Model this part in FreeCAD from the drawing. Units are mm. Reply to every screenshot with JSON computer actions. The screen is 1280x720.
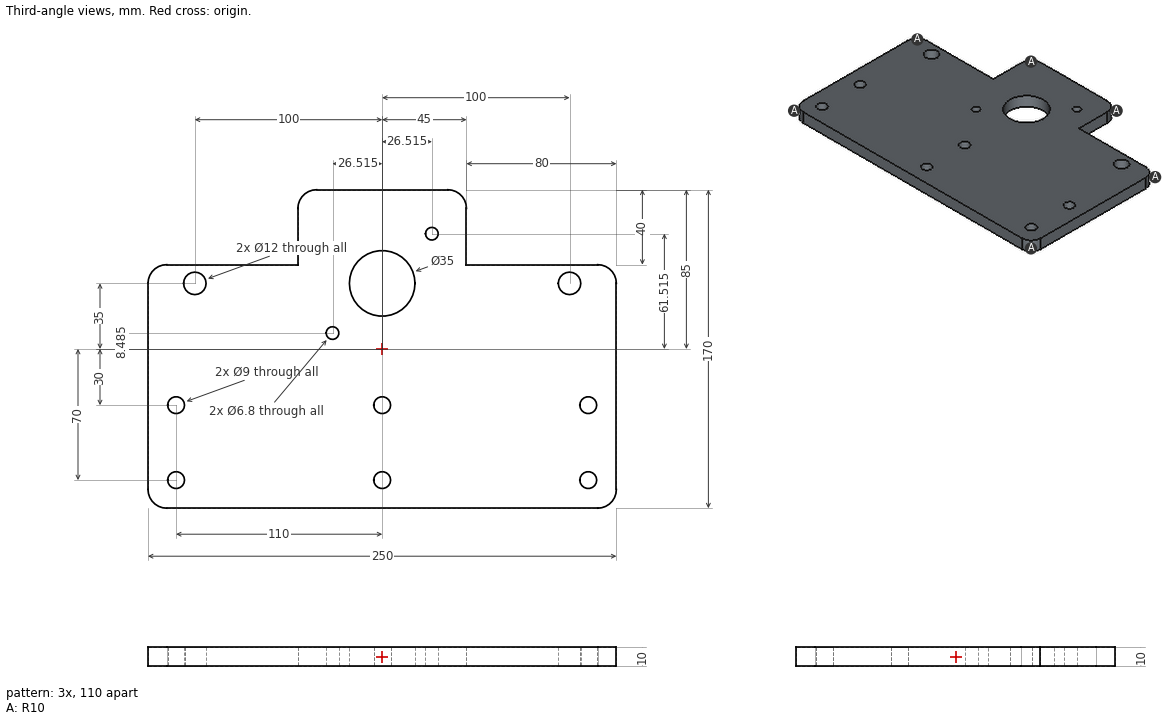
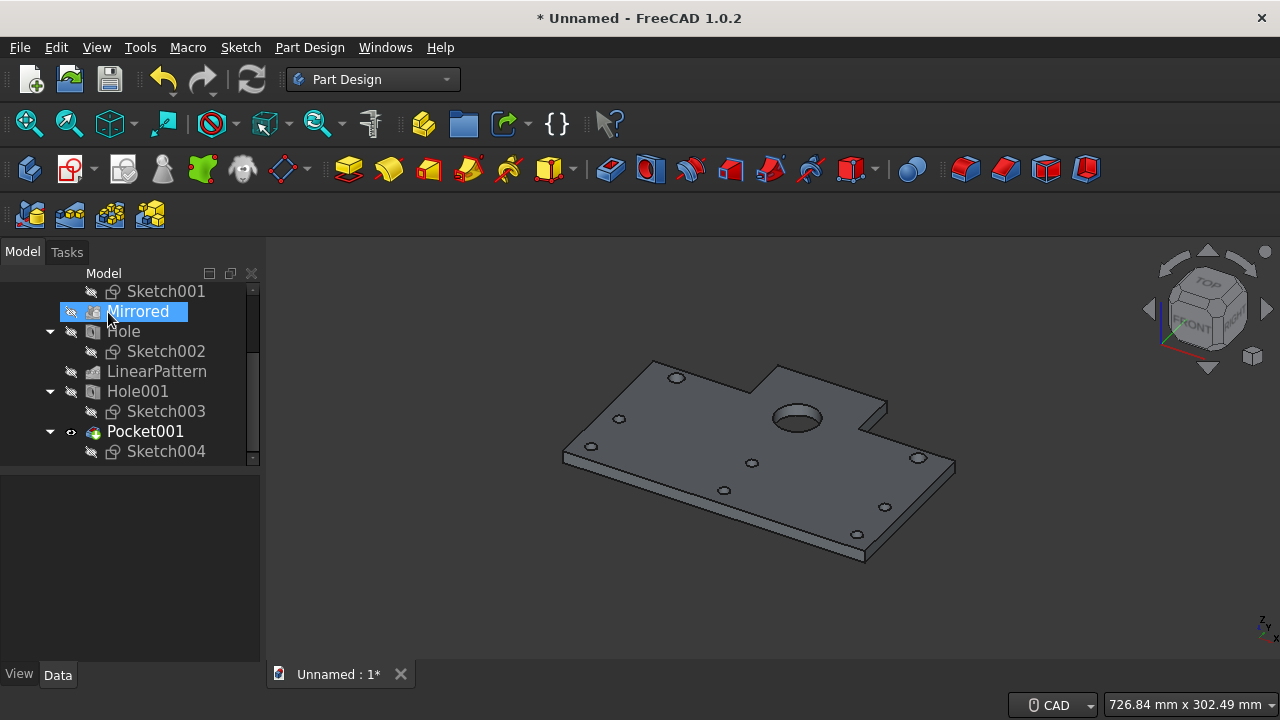
{"action": "left_click", "coordinate": [859, 470]}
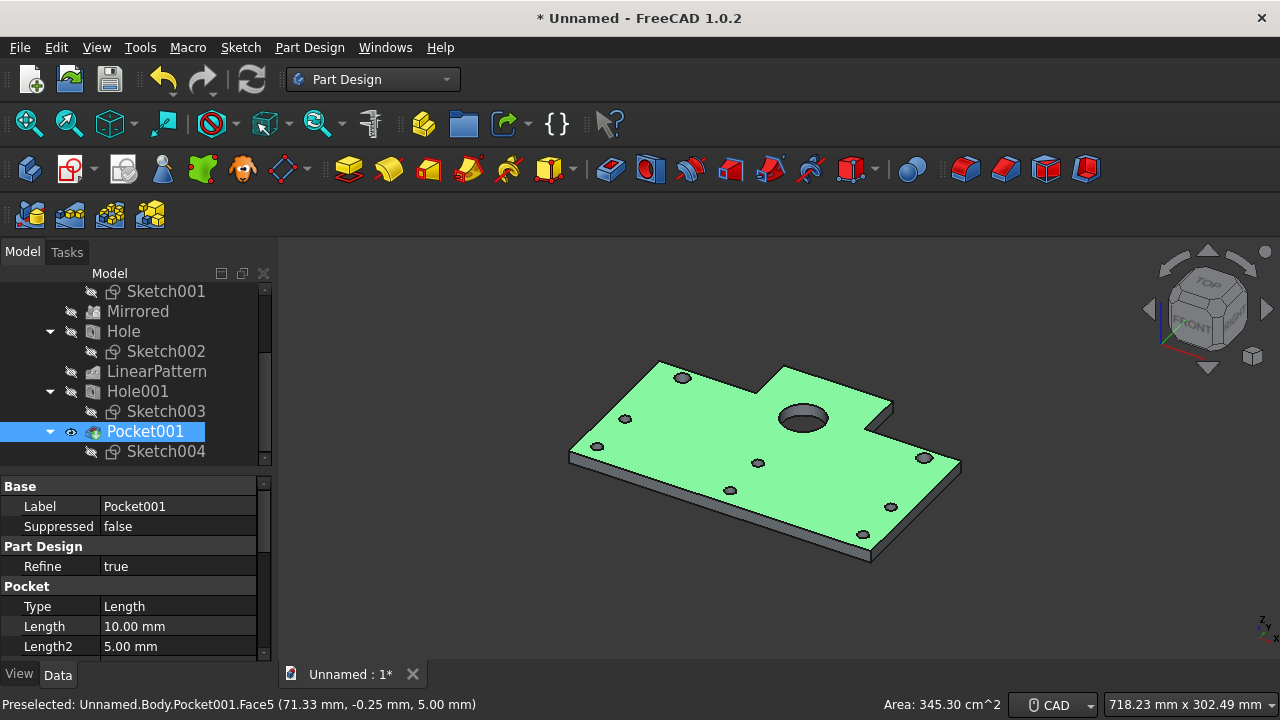
{"action": "left_click", "coordinate": [70, 170]}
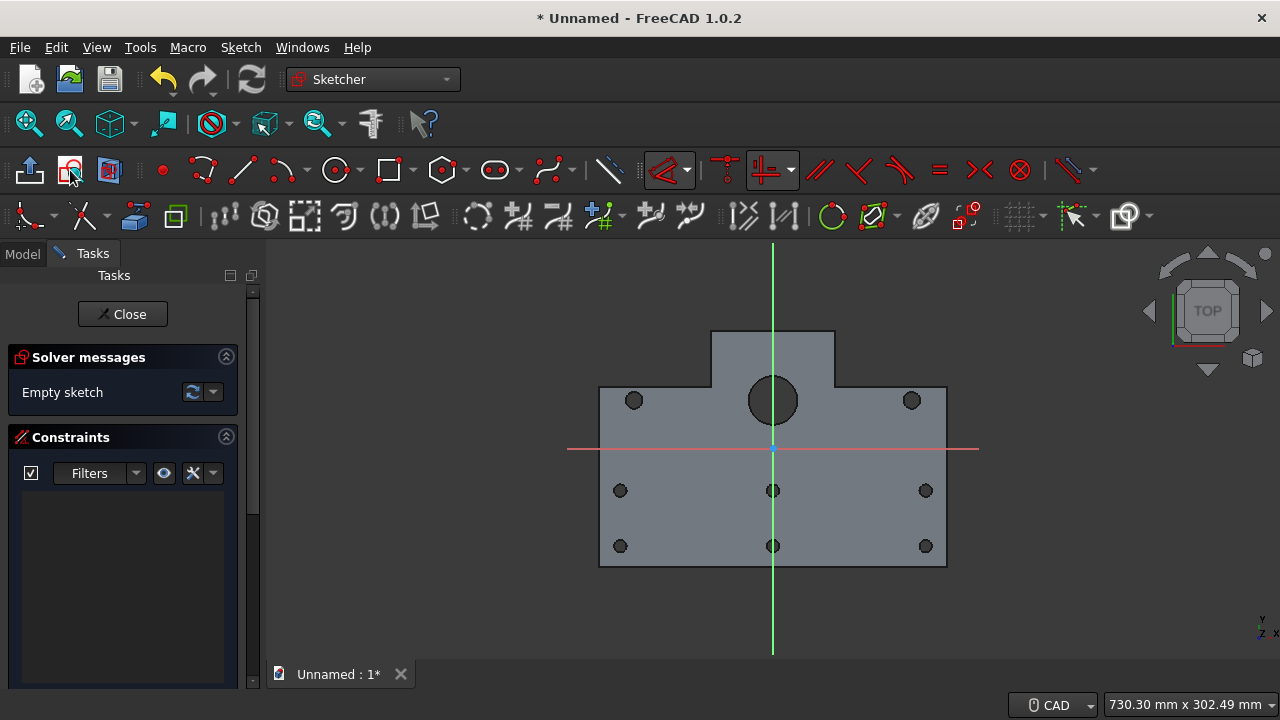
{"action": "scroll", "coordinate": [813, 378], "scroll_direction": "up", "scroll_amount": 5}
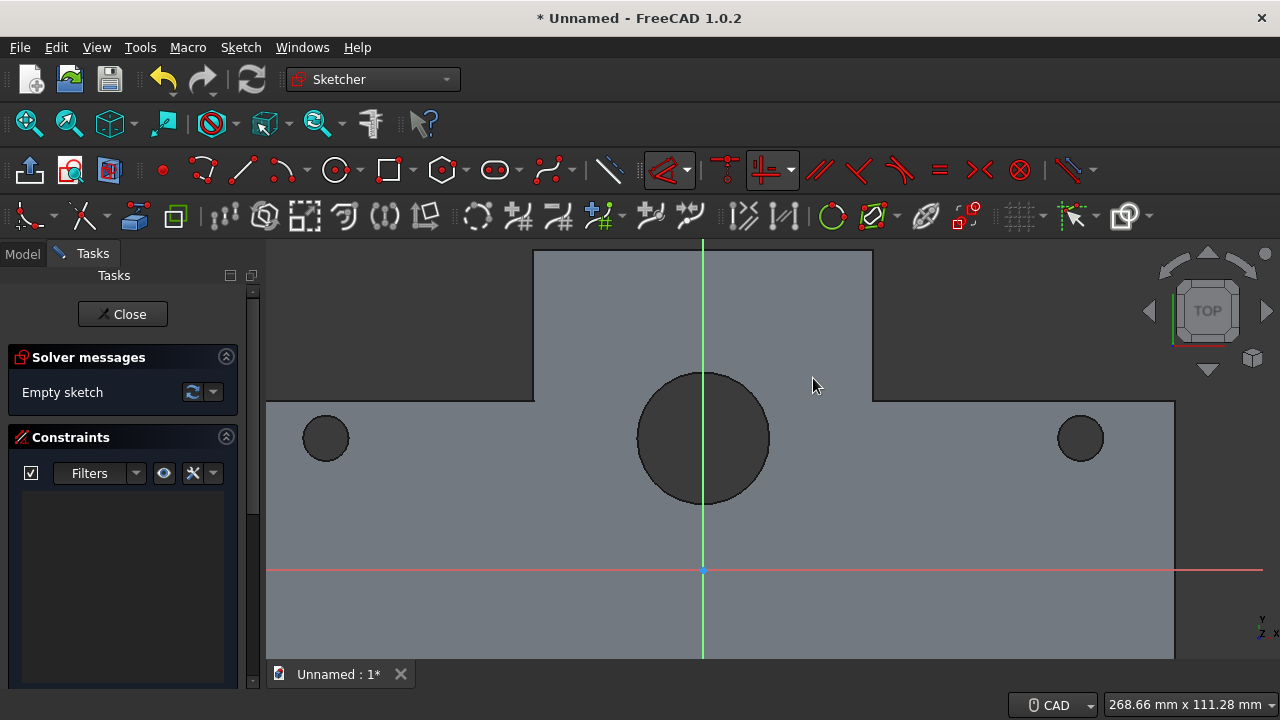
{"action": "left_click", "coordinate": [336, 170]}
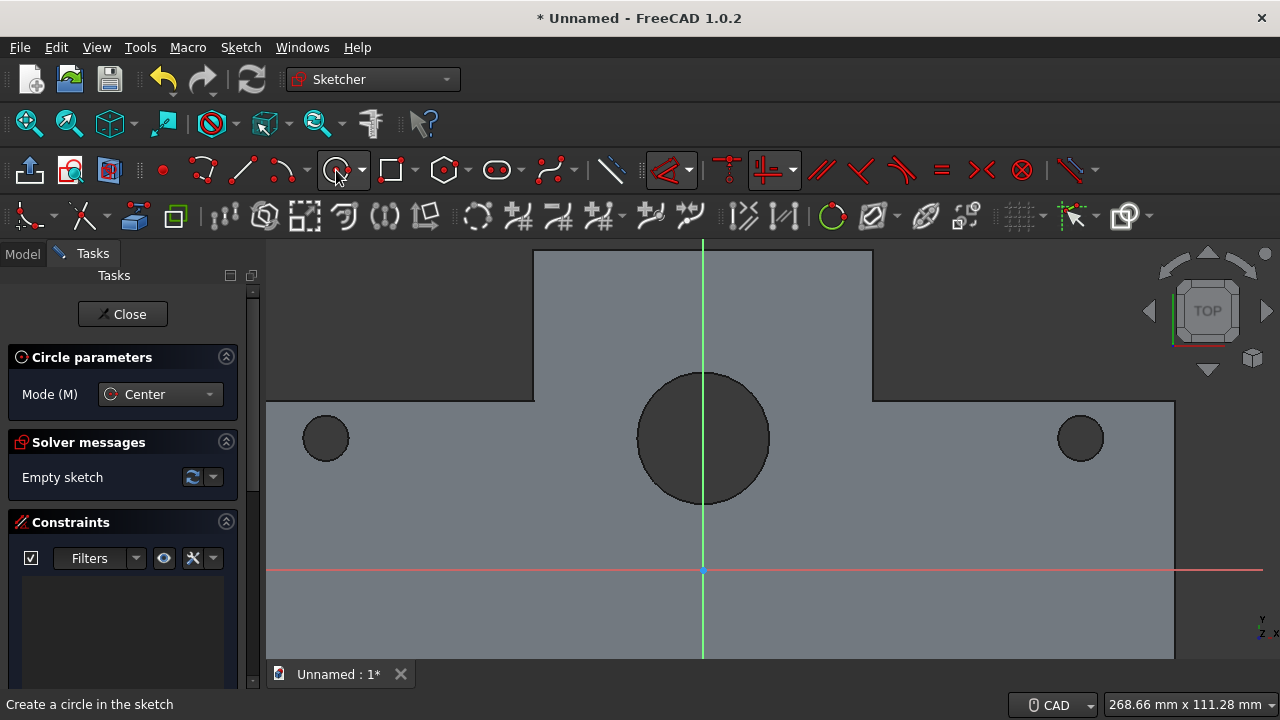
{"action": "scroll", "coordinate": [603, 538], "scroll_direction": "up", "scroll_amount": 3}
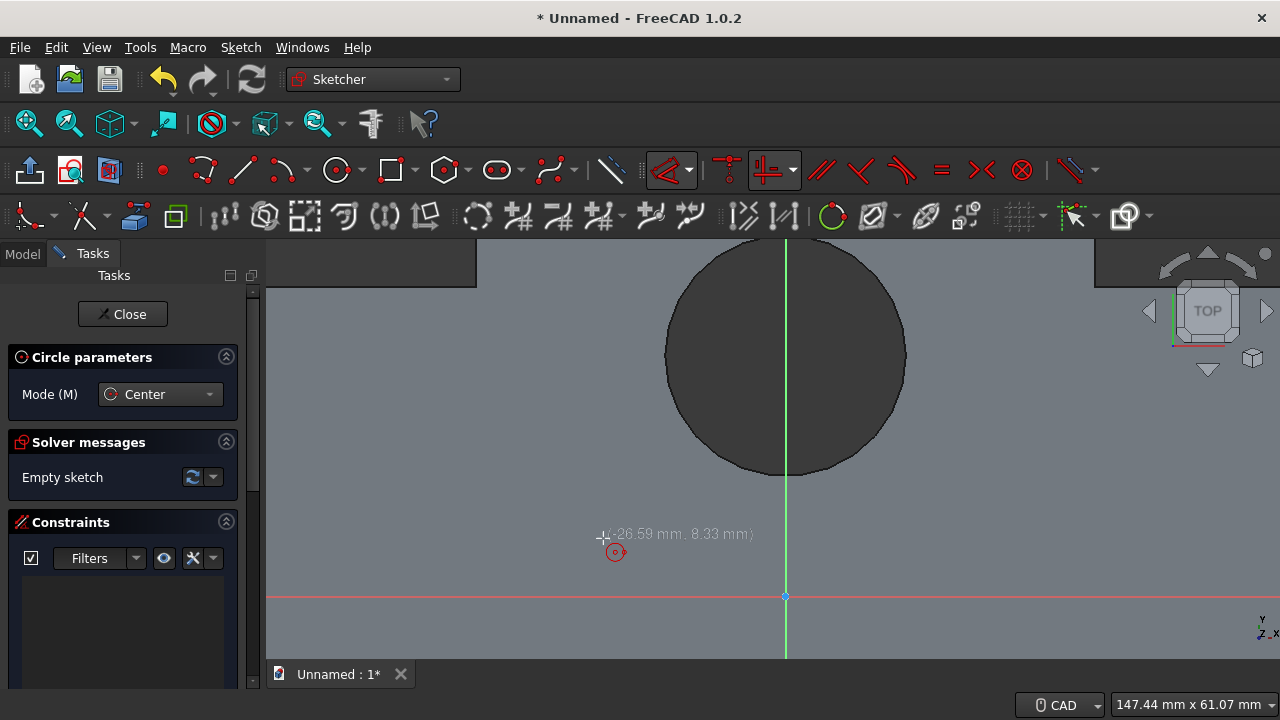
{"action": "left_click", "coordinate": [603, 538]}
{"action": "mouse_move", "coordinate": [620, 522]}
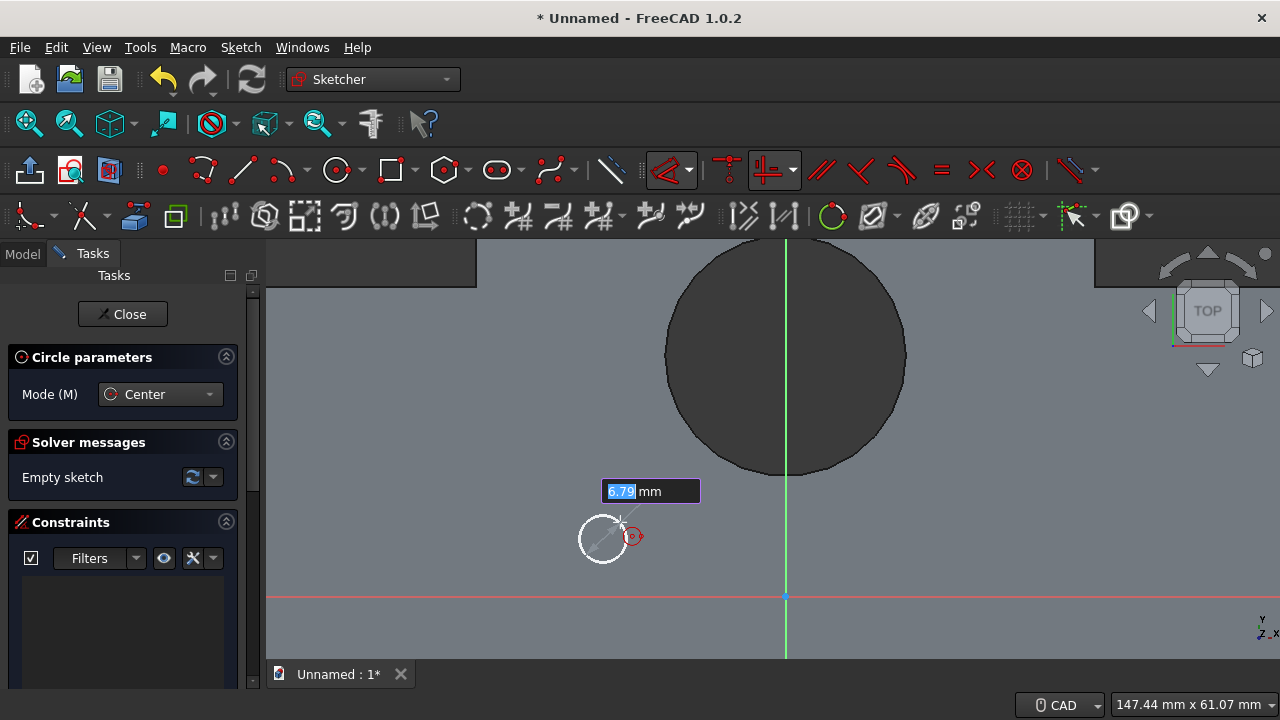
{"action": "type", "text": "6.8"}
{"action": "key", "text": "Return"}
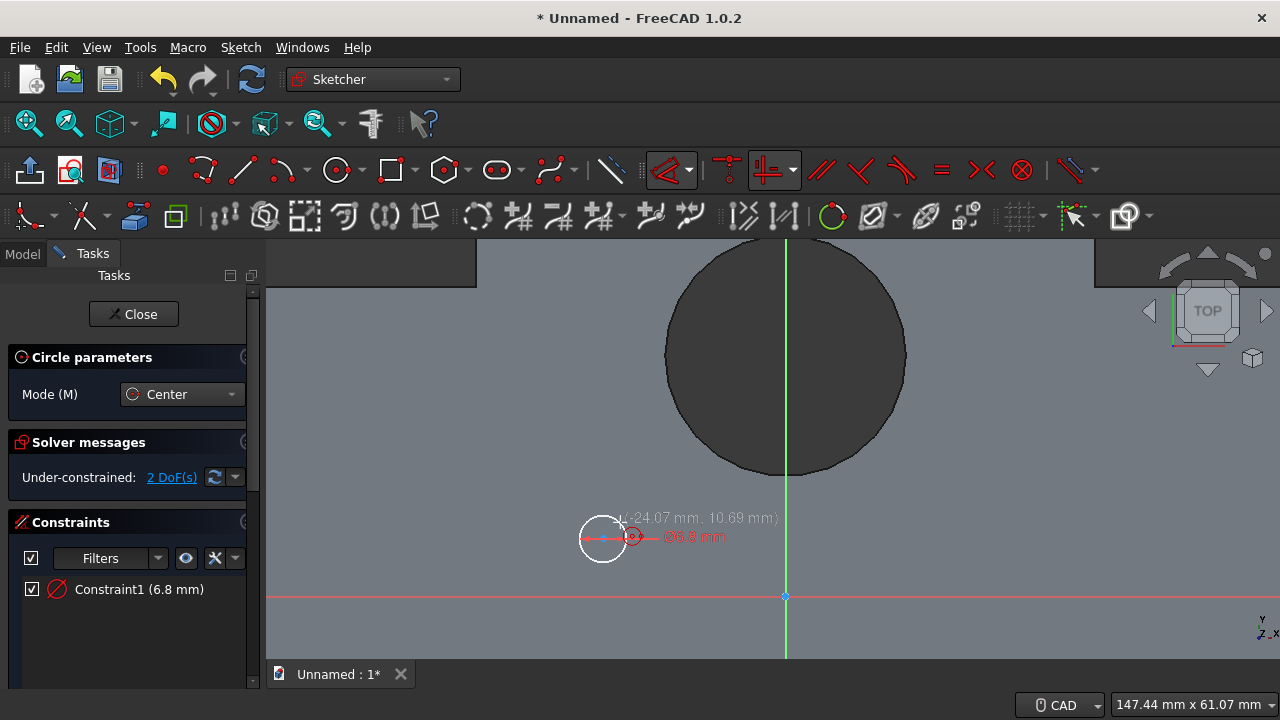
{"action": "scroll", "coordinate": [606, 541], "scroll_direction": "down", "scroll_amount": 3}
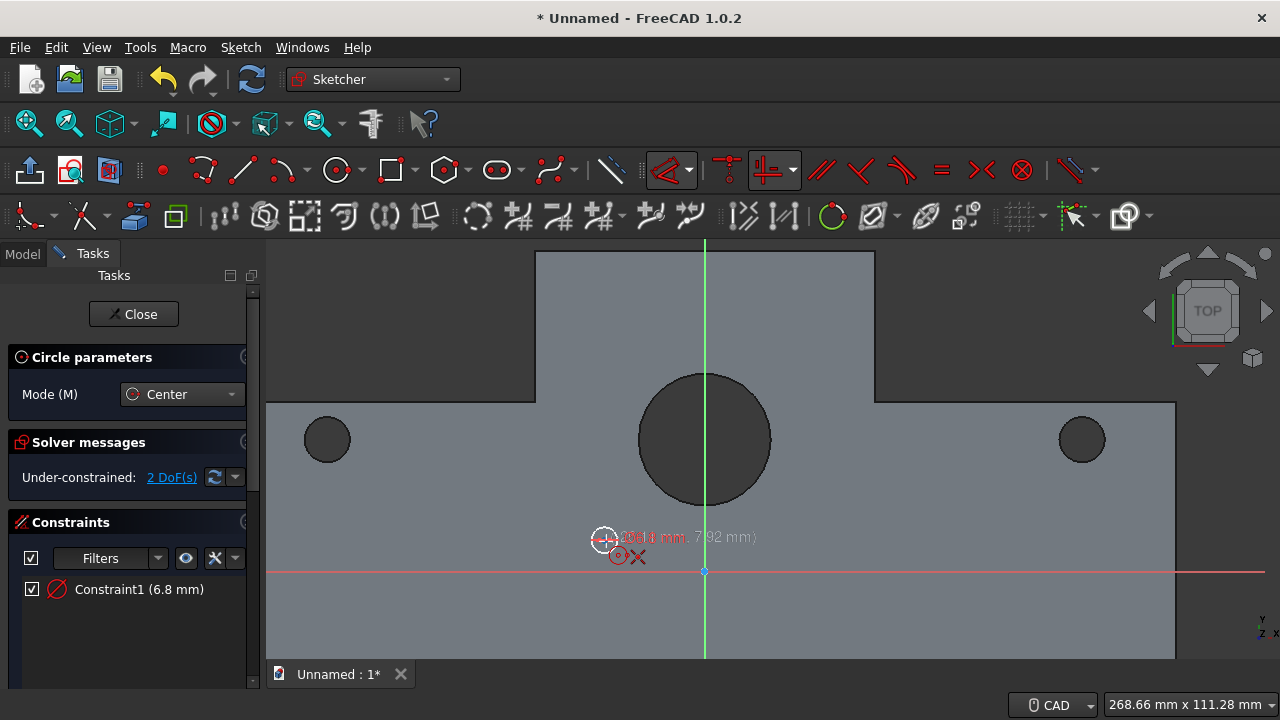
{"action": "scroll", "coordinate": [805, 340], "scroll_direction": "up", "scroll_amount": 3}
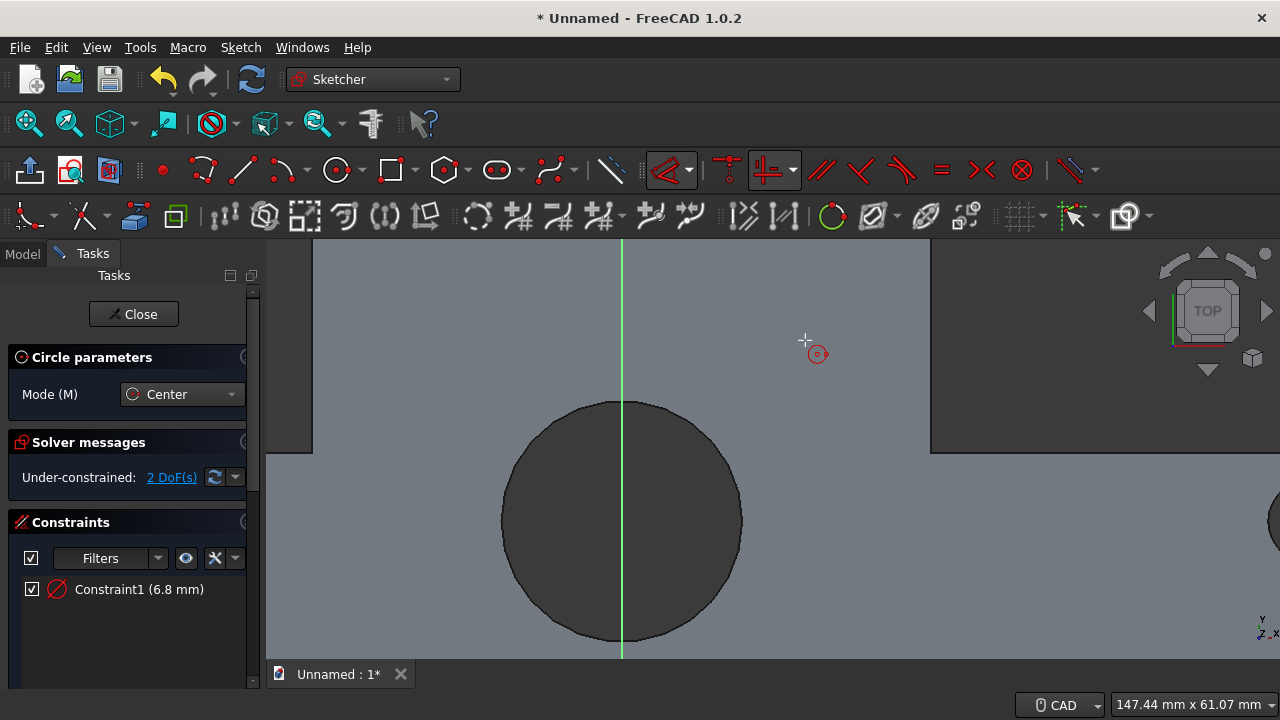
{"action": "left_click", "coordinate": [804, 339]}
{"action": "mouse_move", "coordinate": [821, 323]}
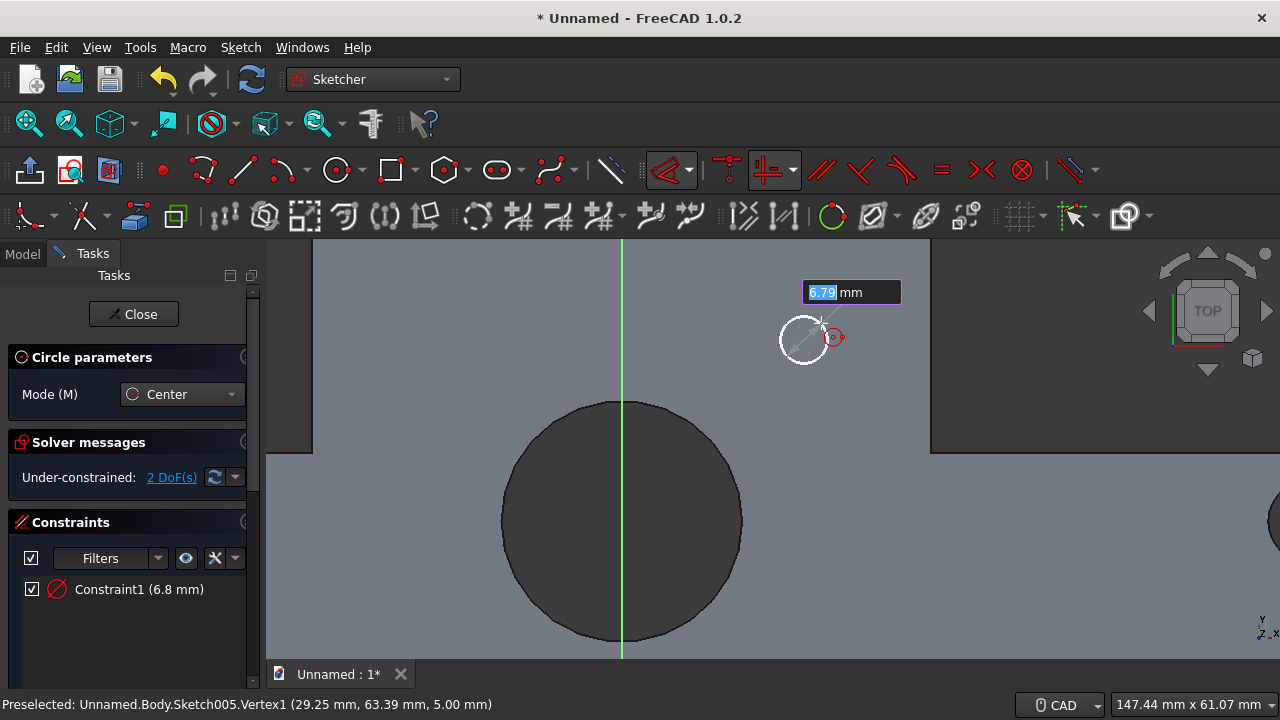
{"action": "type", "text": "6.8"}
{"action": "key", "text": "Return"}
{"action": "key", "text": "Escape"}